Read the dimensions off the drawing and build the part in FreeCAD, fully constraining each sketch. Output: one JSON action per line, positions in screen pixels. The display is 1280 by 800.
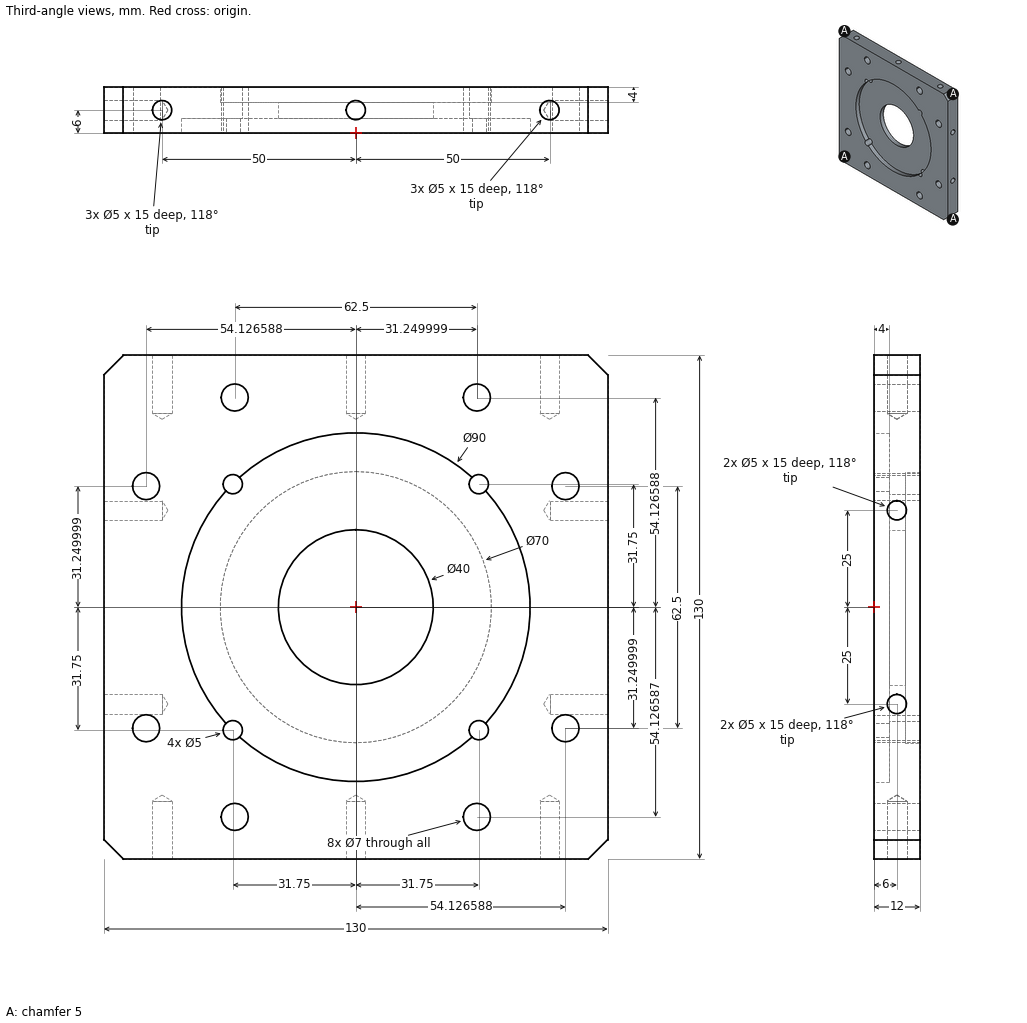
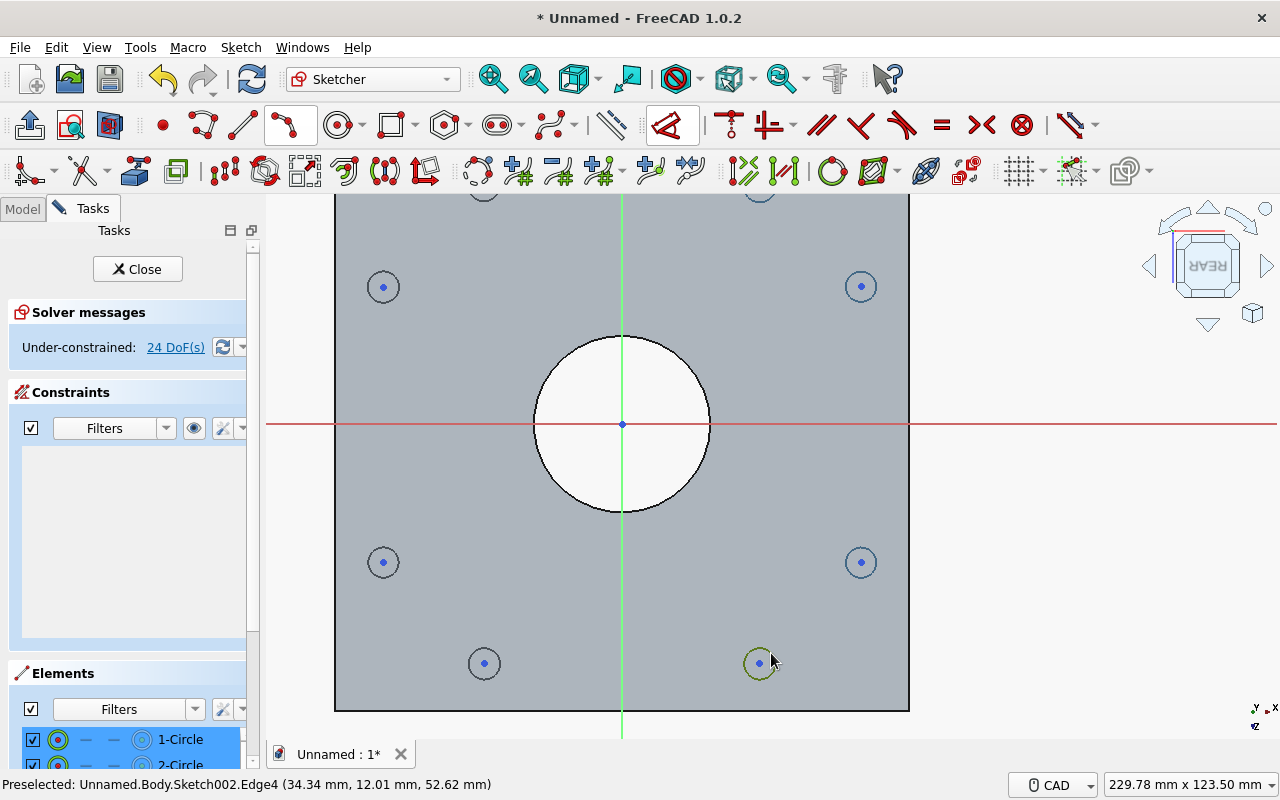
{"action": "left_click", "coordinate": [495, 653]}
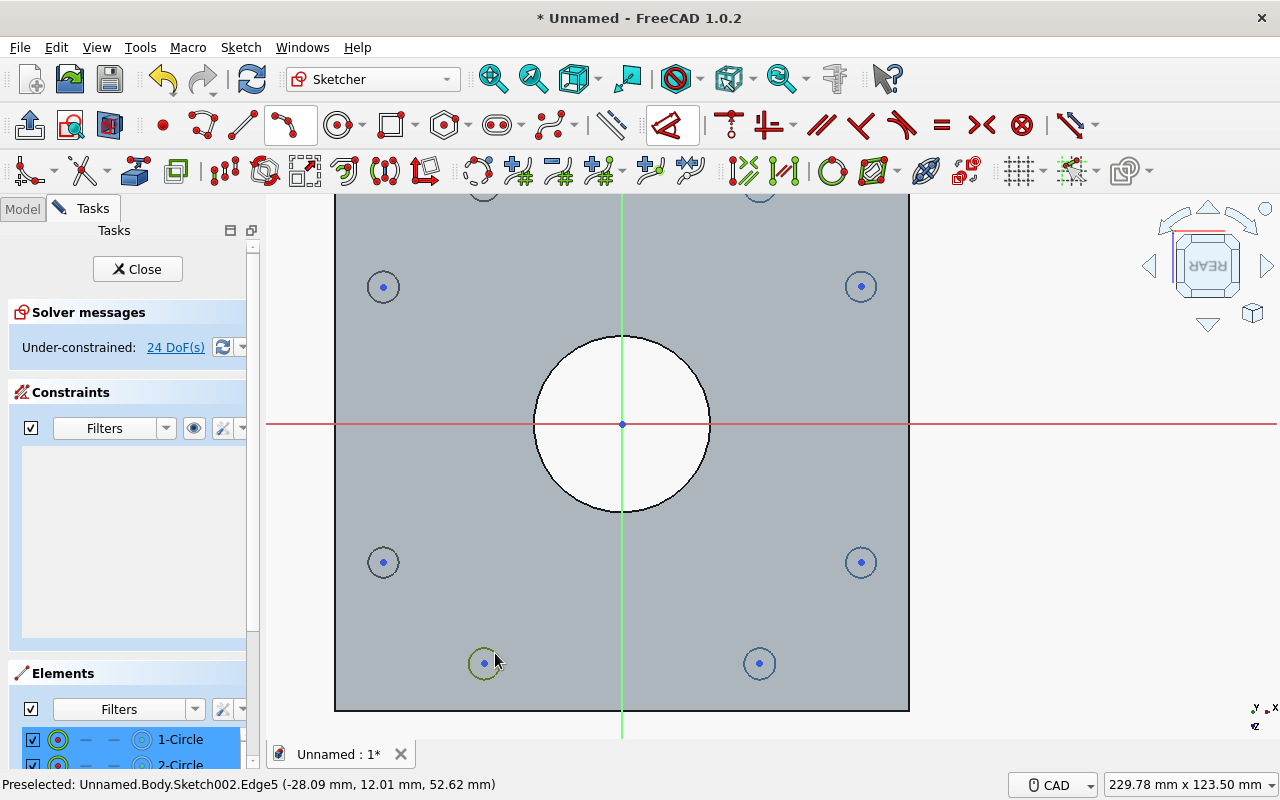
{"action": "left_click", "coordinate": [394, 552]}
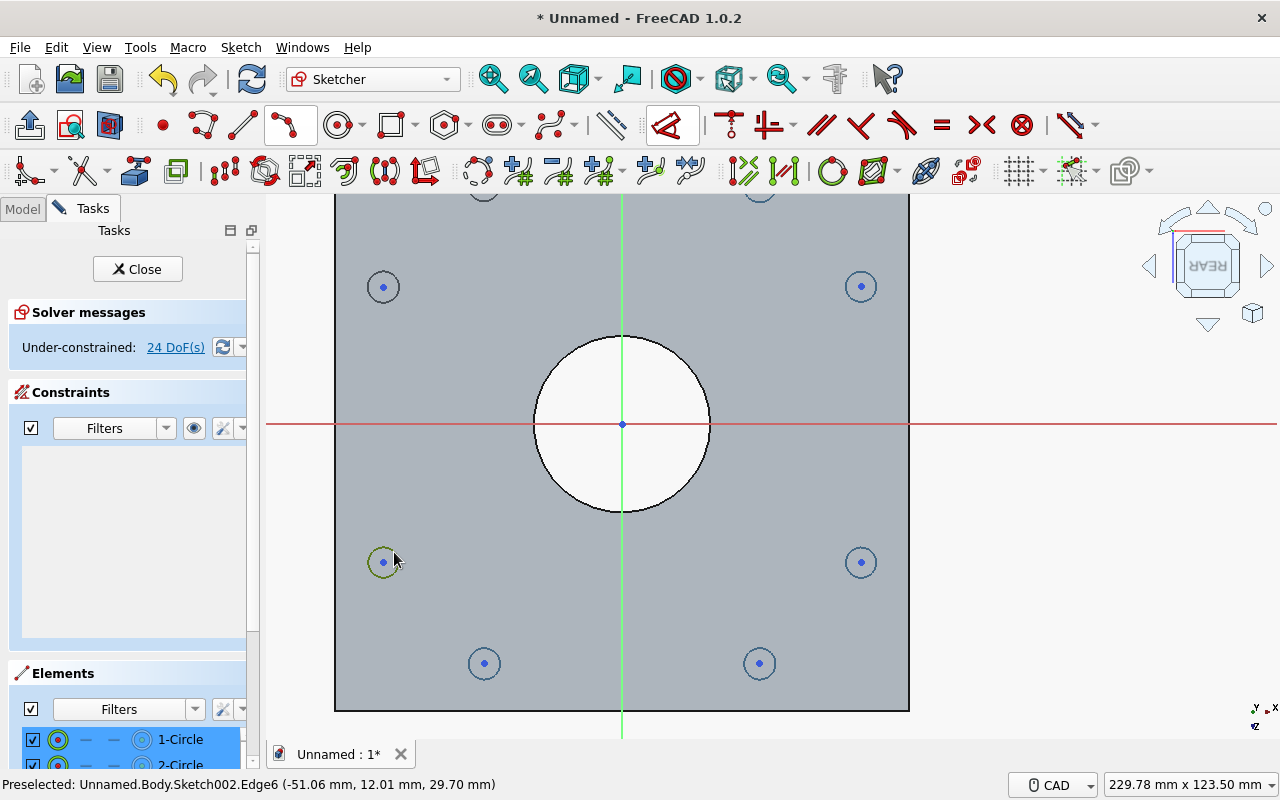
{"action": "left_click", "coordinate": [394, 276]}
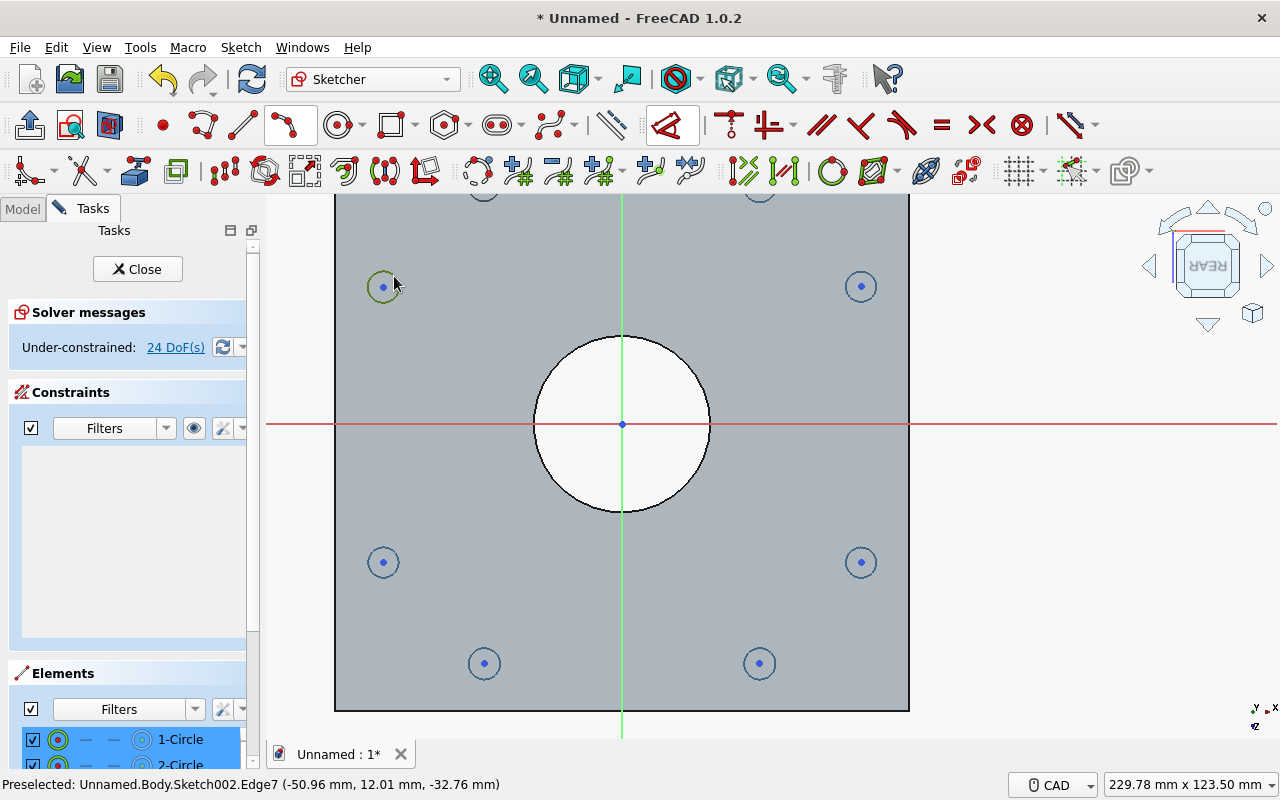
{"action": "scroll", "coordinate": [872, 553], "scroll_direction": "down", "scroll_amount": 2}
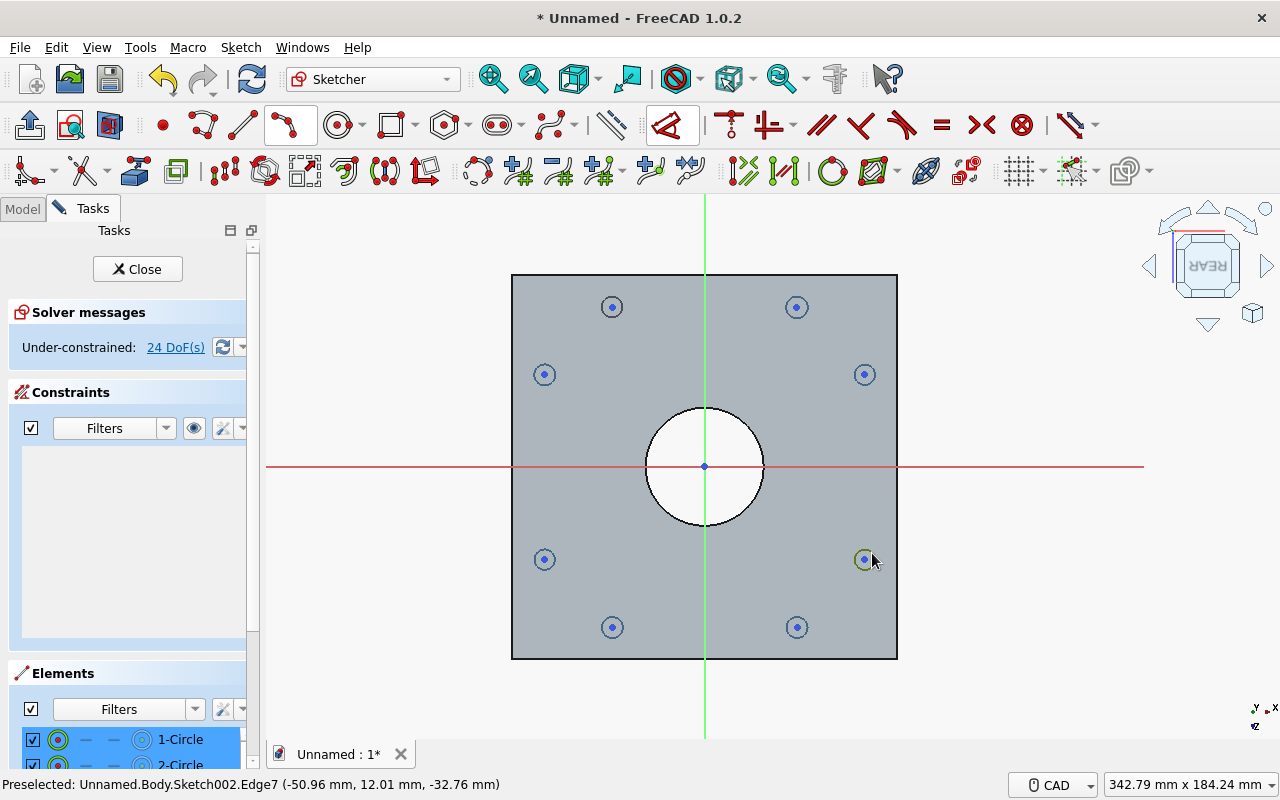
{"action": "scroll", "coordinate": [619, 300], "scroll_direction": "up", "scroll_amount": 2}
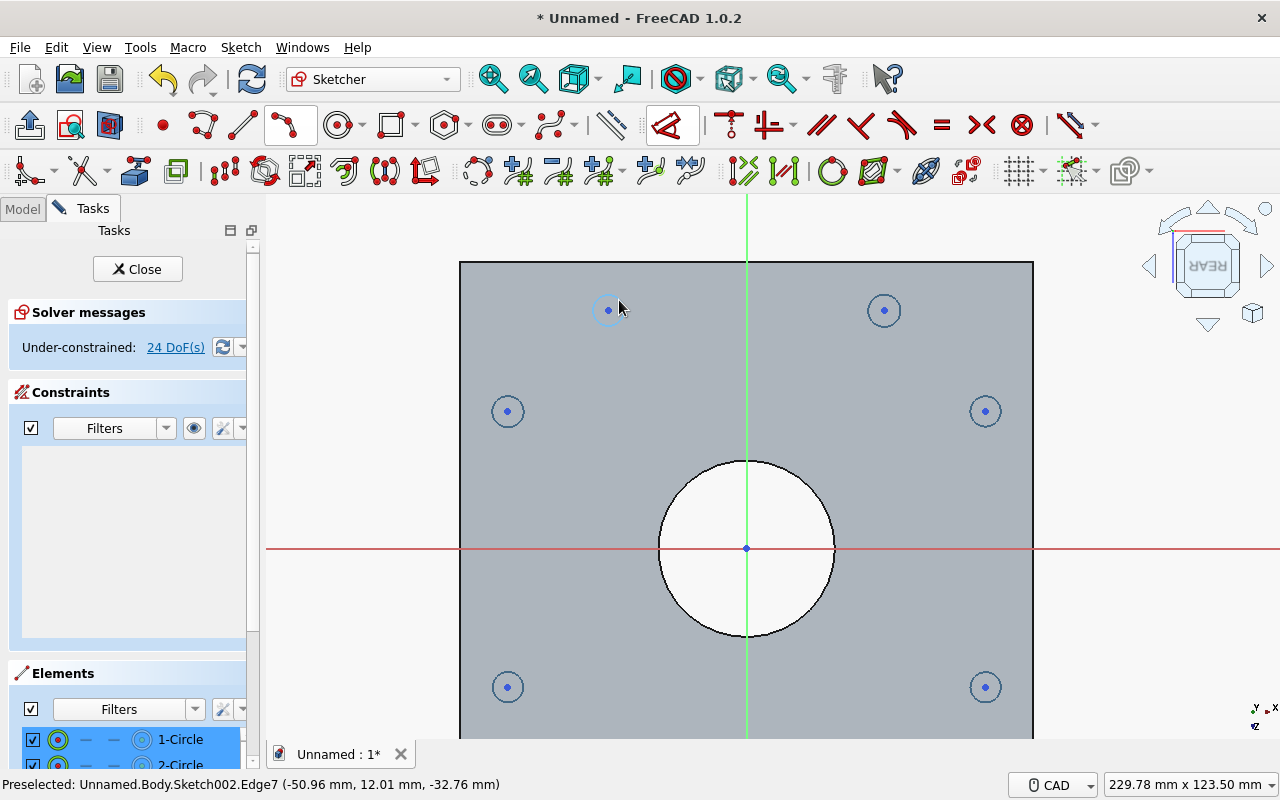
{"action": "left_click", "coordinate": [619, 300]}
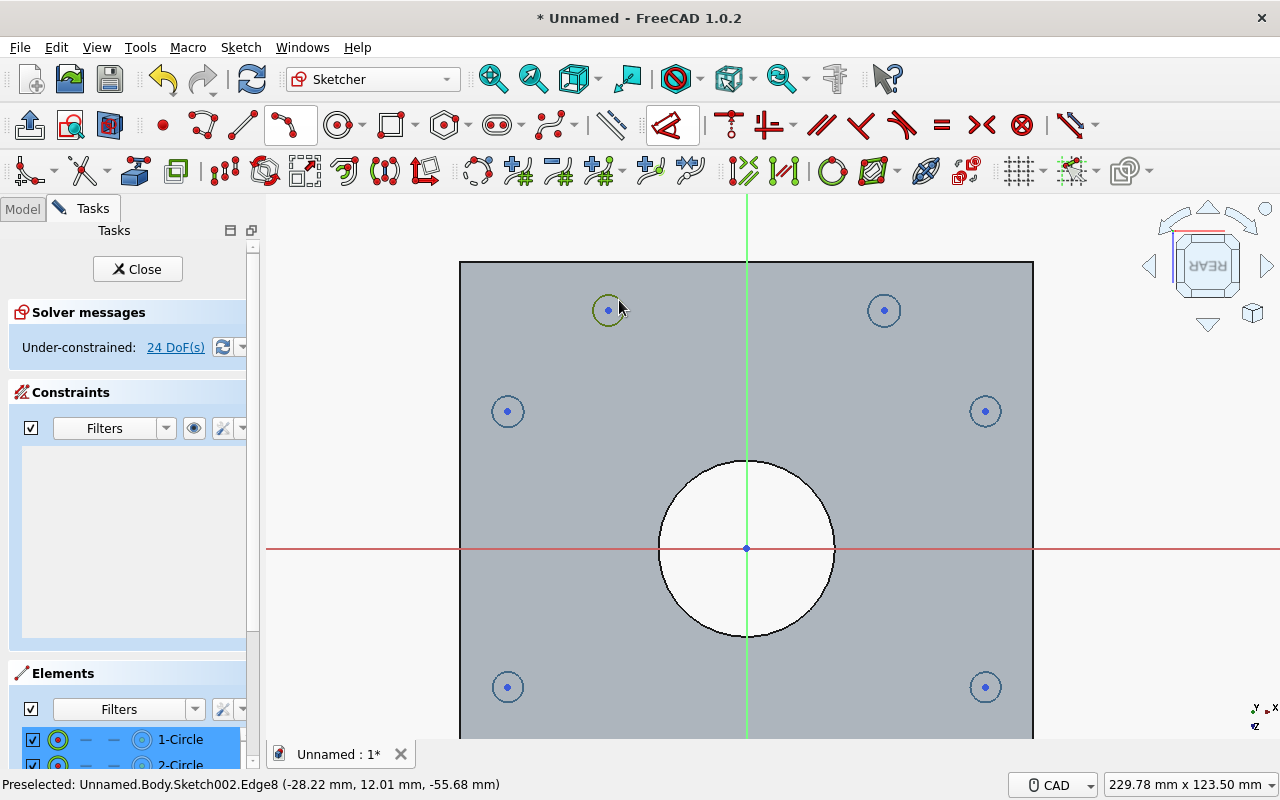
{"action": "key", "text": "e"}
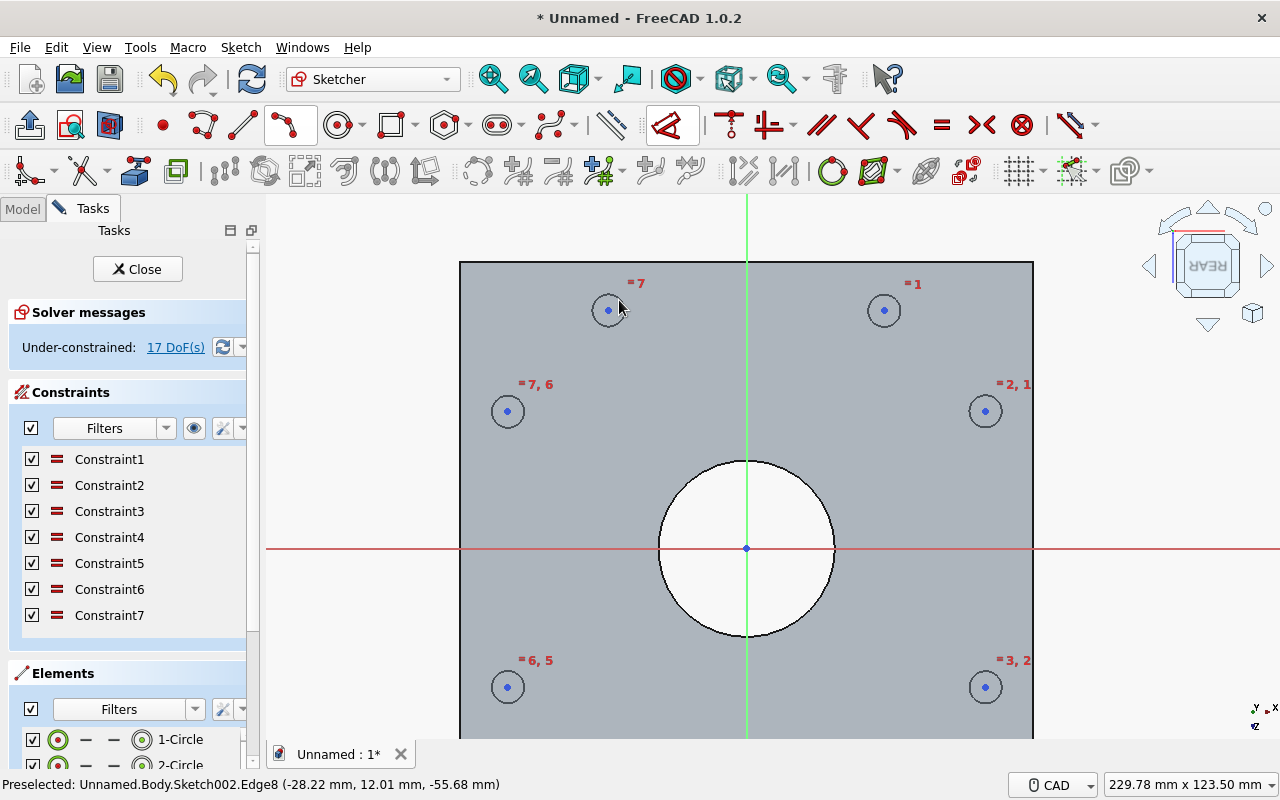
{"action": "left_click", "coordinate": [986, 411]}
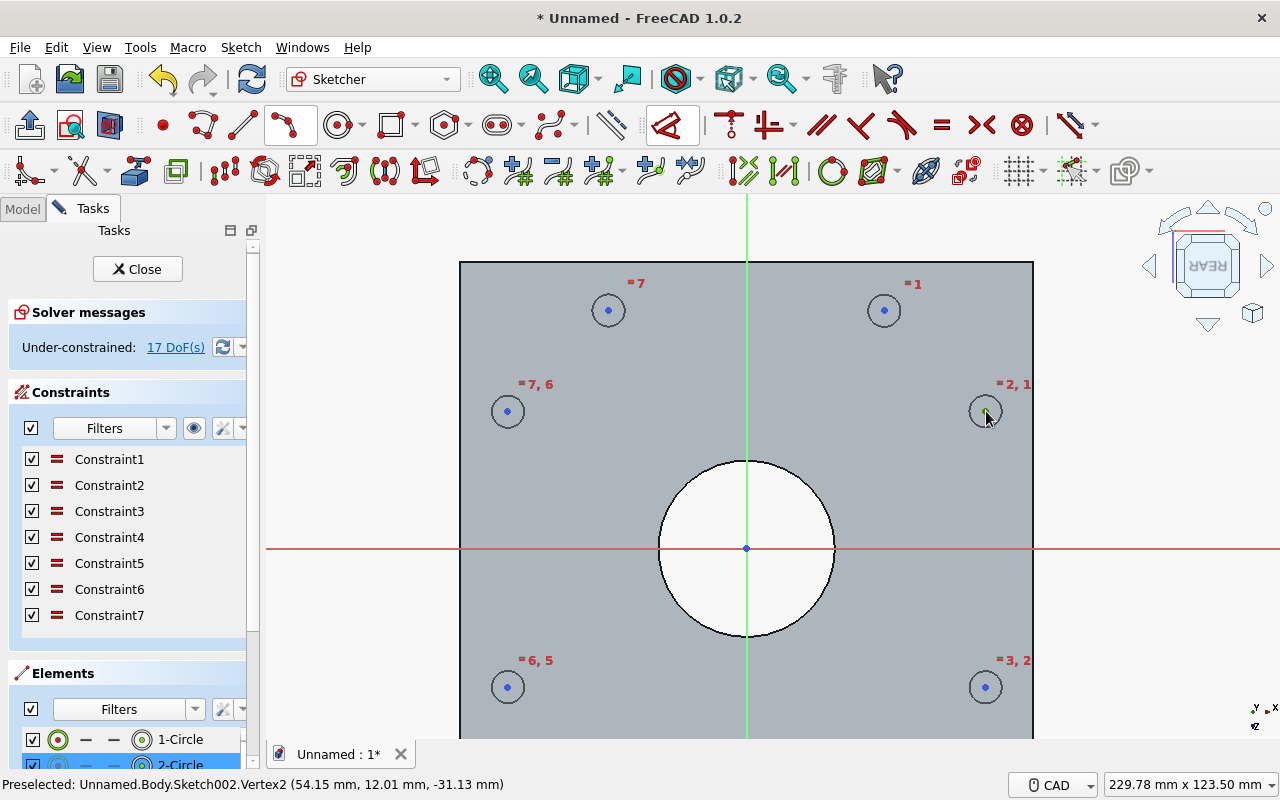
{"action": "left_click", "coordinate": [986, 687]}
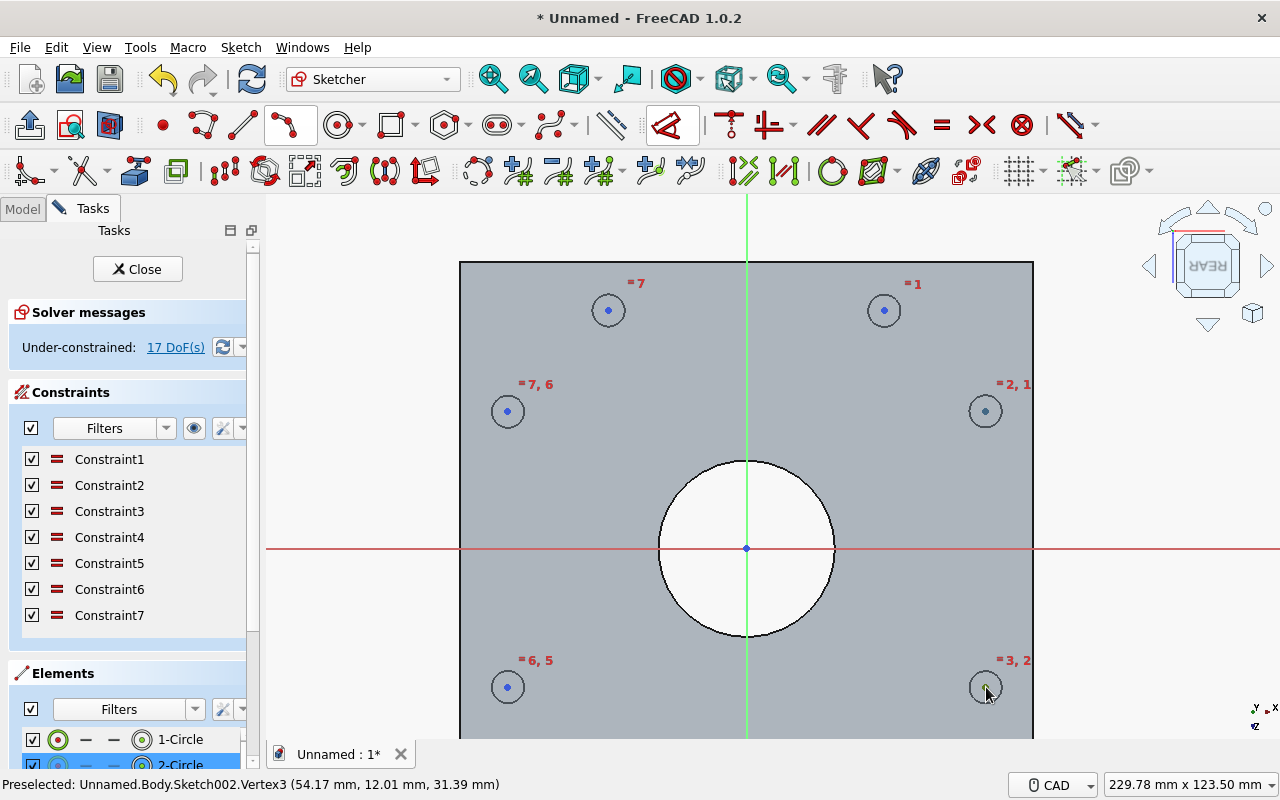
{"action": "key", "text": "v"}